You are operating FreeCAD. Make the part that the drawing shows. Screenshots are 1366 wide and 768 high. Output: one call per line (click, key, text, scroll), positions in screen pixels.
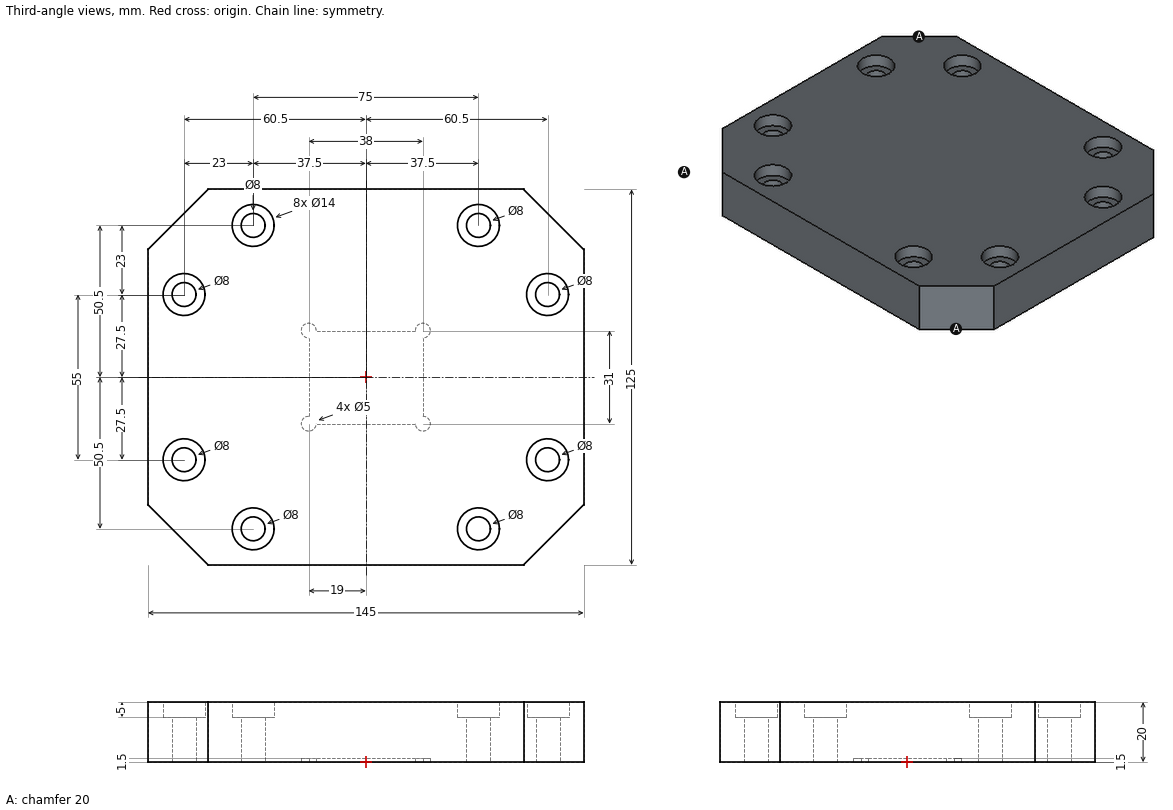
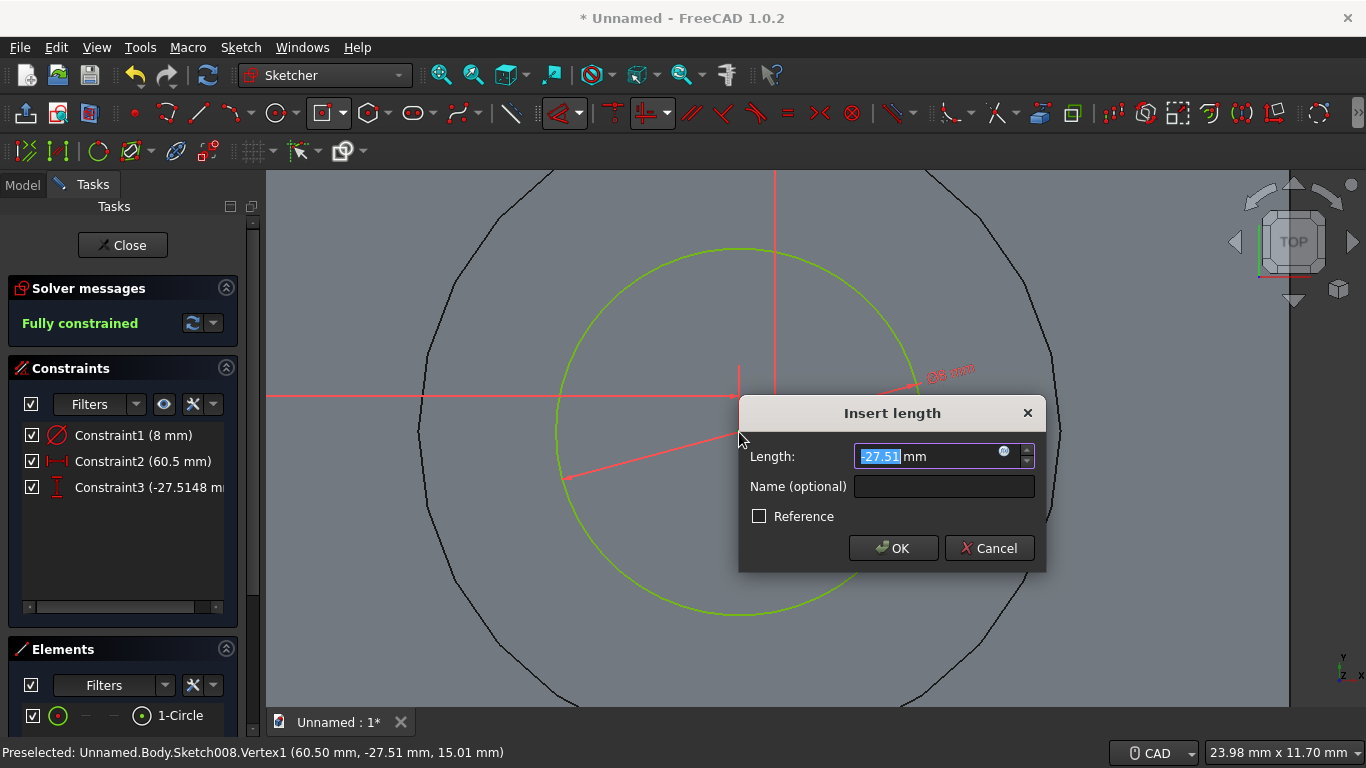
text(-27.5)
key(Return)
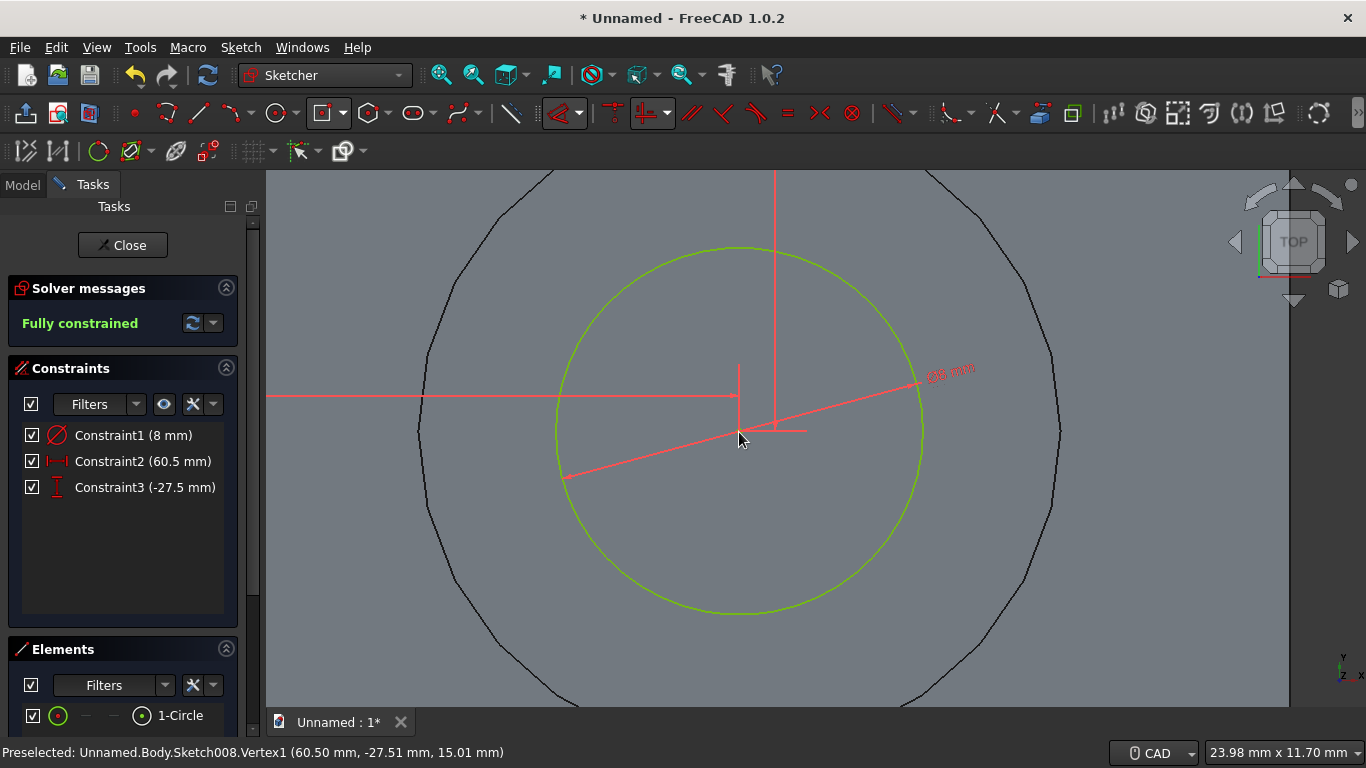
click(123, 245)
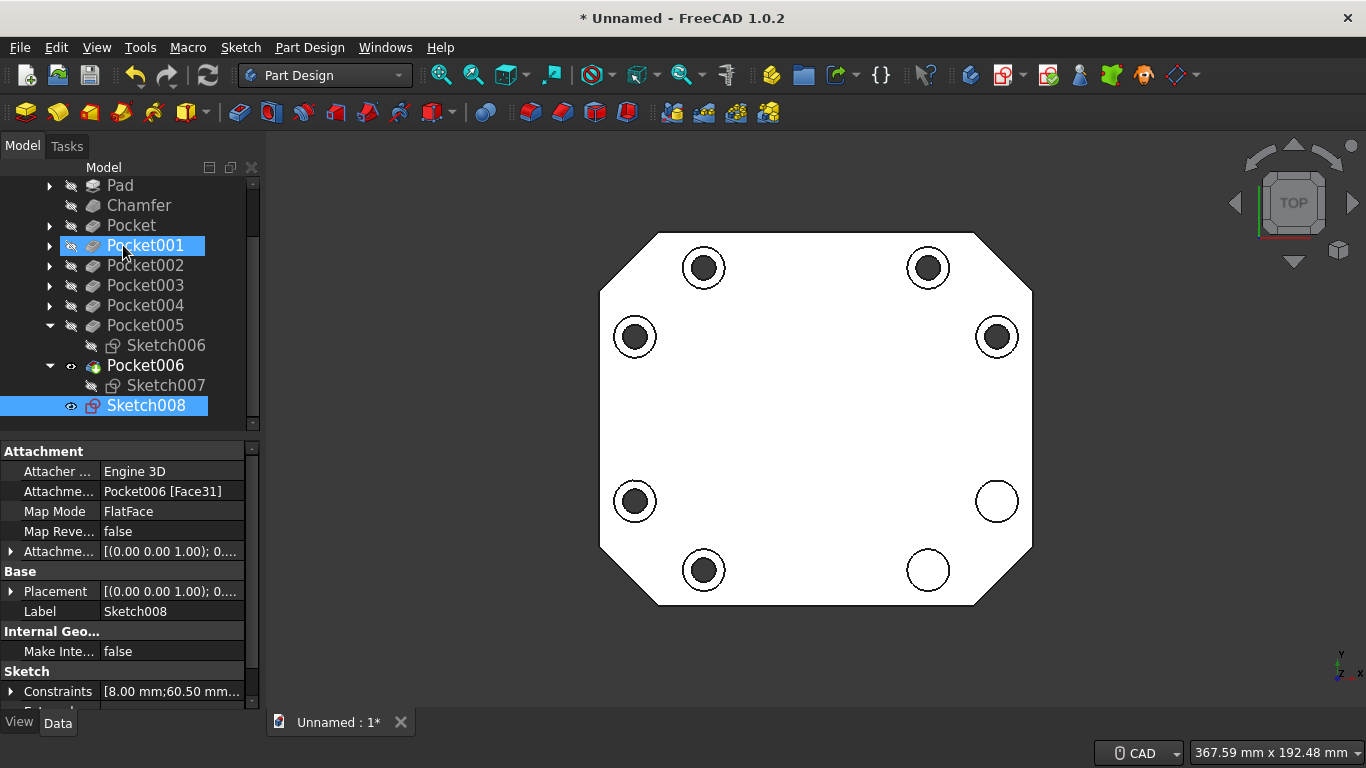
click(240, 112)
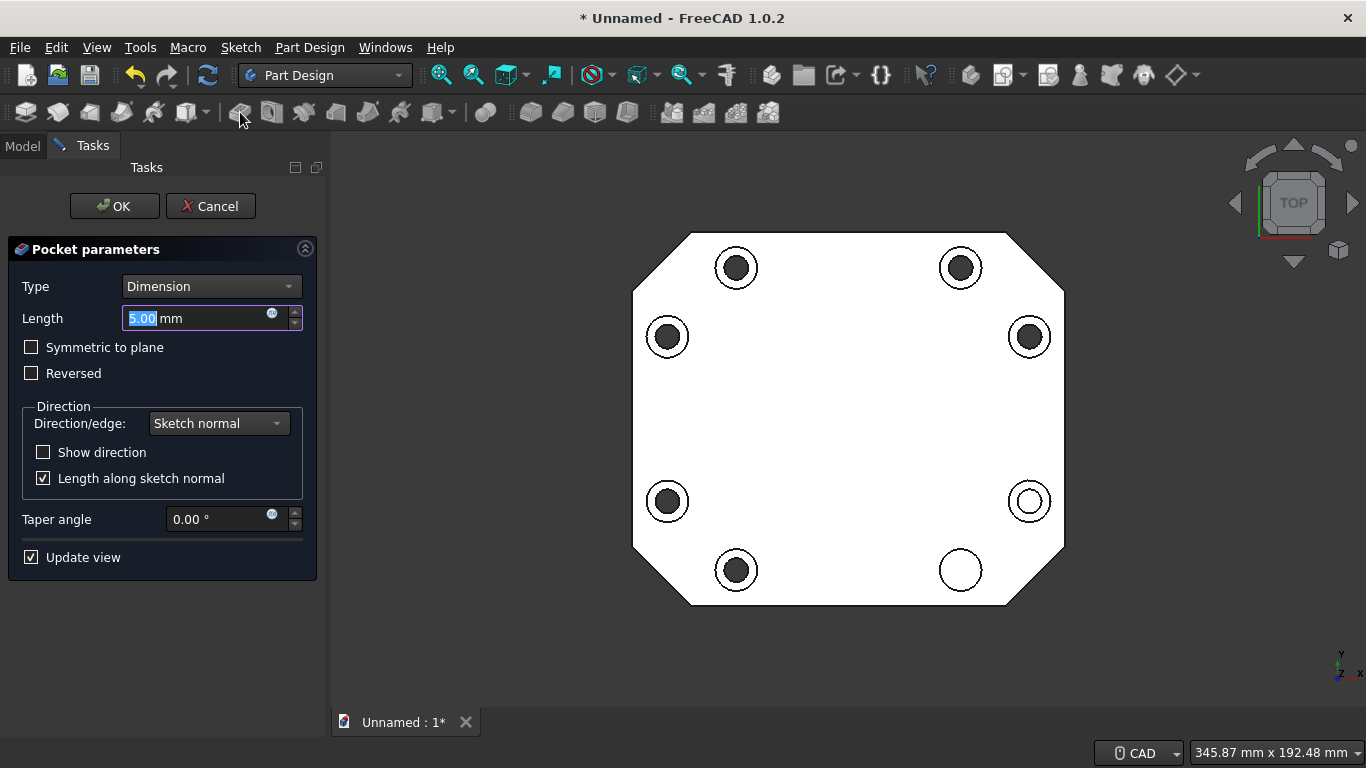
click(212, 286)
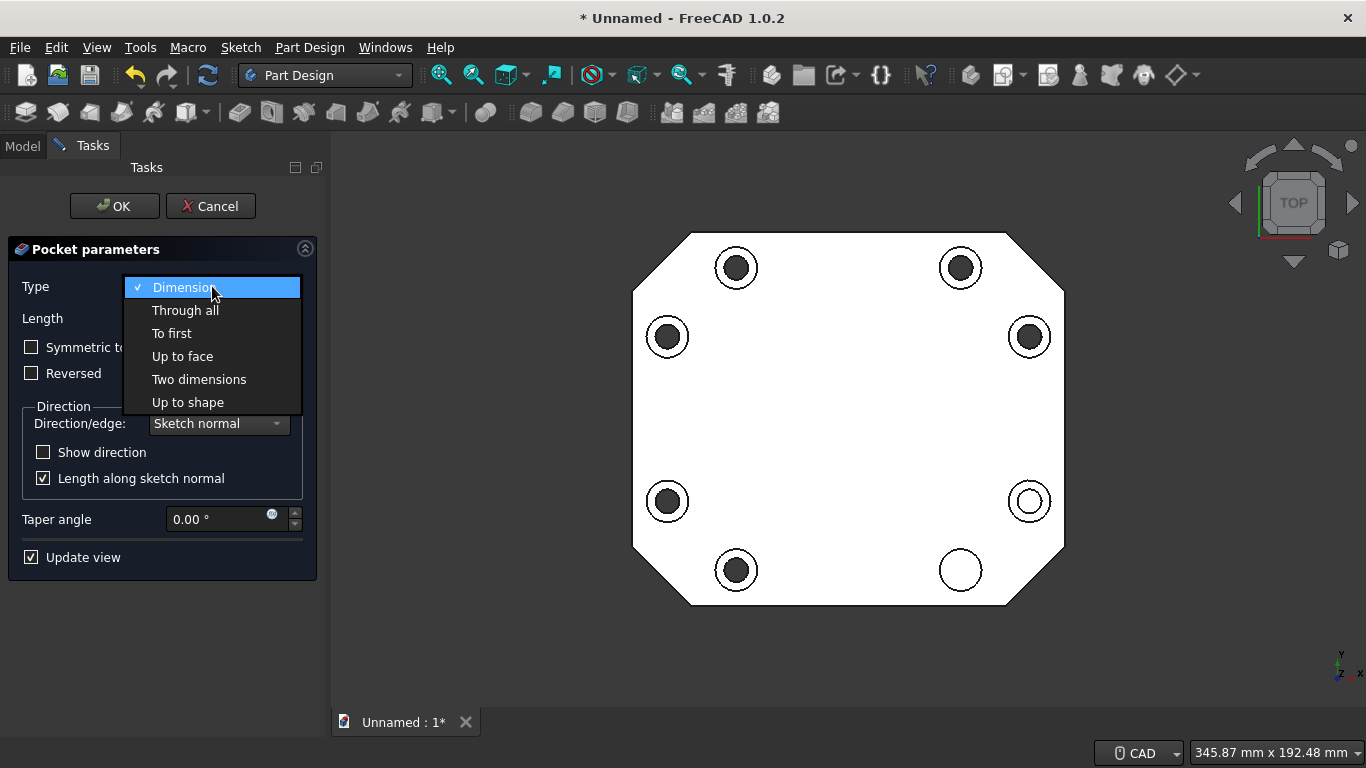
click(212, 334)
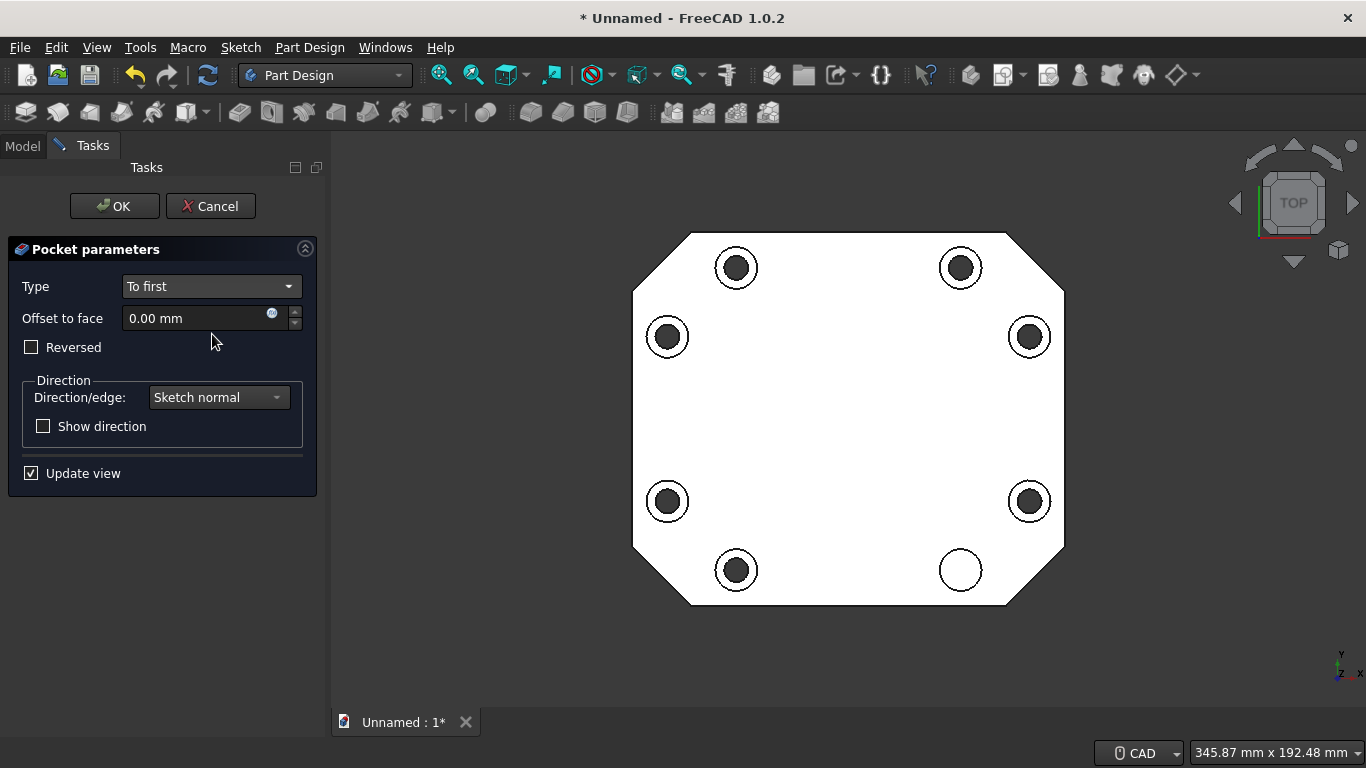
click(115, 206)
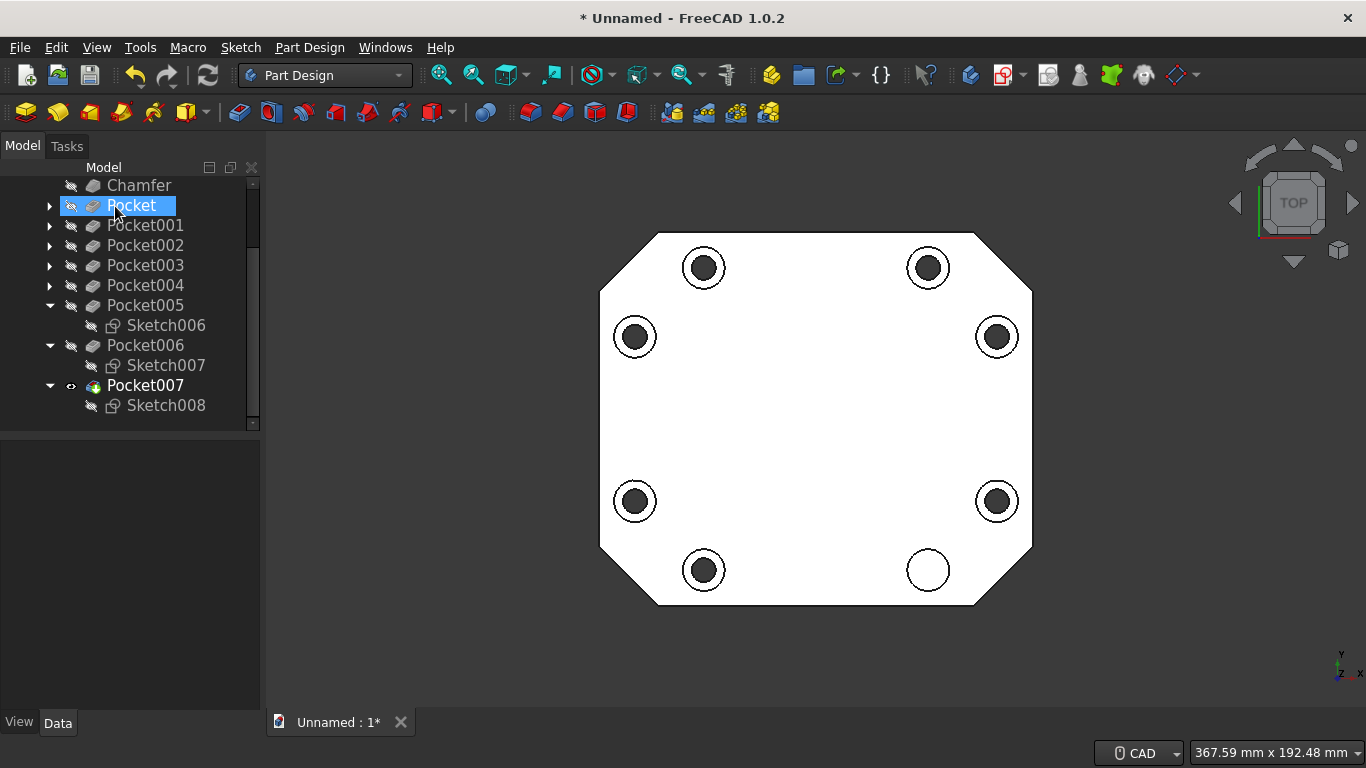
click(928, 569)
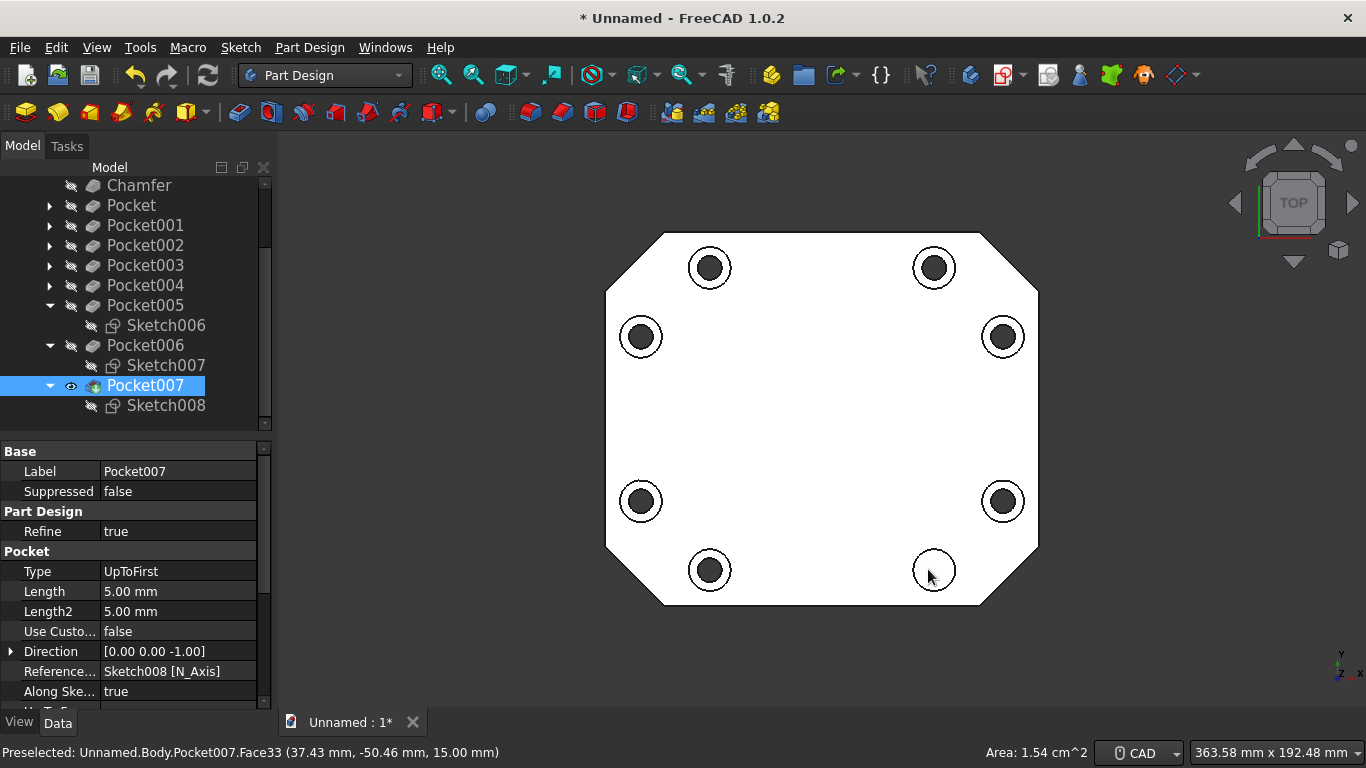
click(1004, 76)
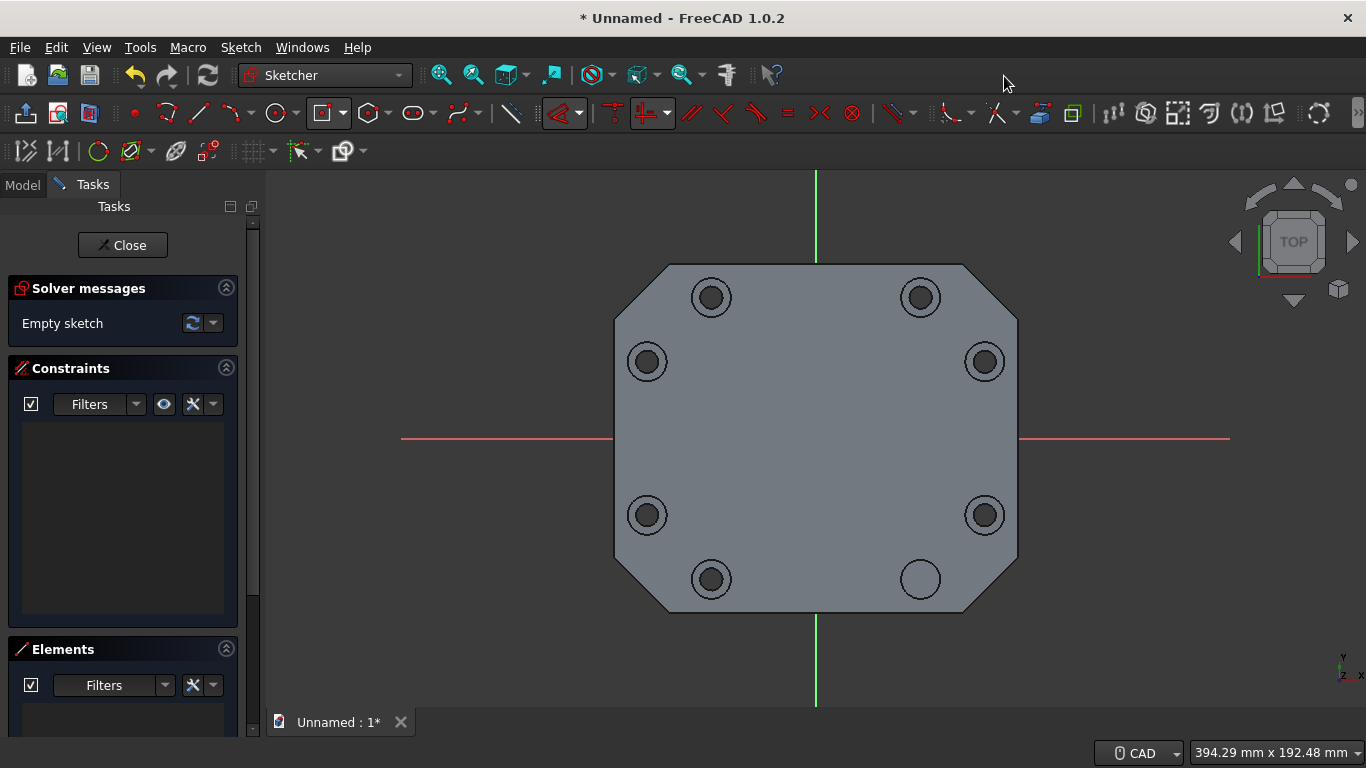
scroll(932, 589, up, 14)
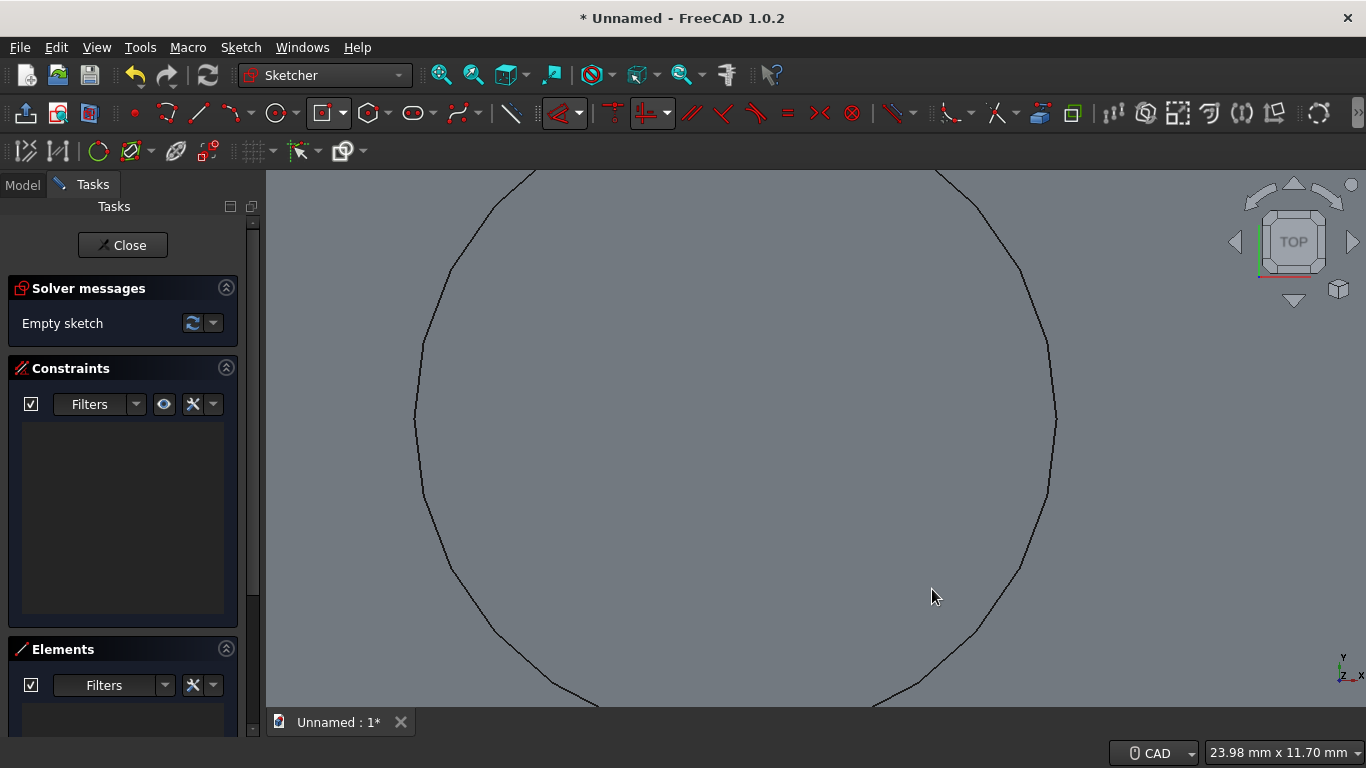
key(g)
key(c)